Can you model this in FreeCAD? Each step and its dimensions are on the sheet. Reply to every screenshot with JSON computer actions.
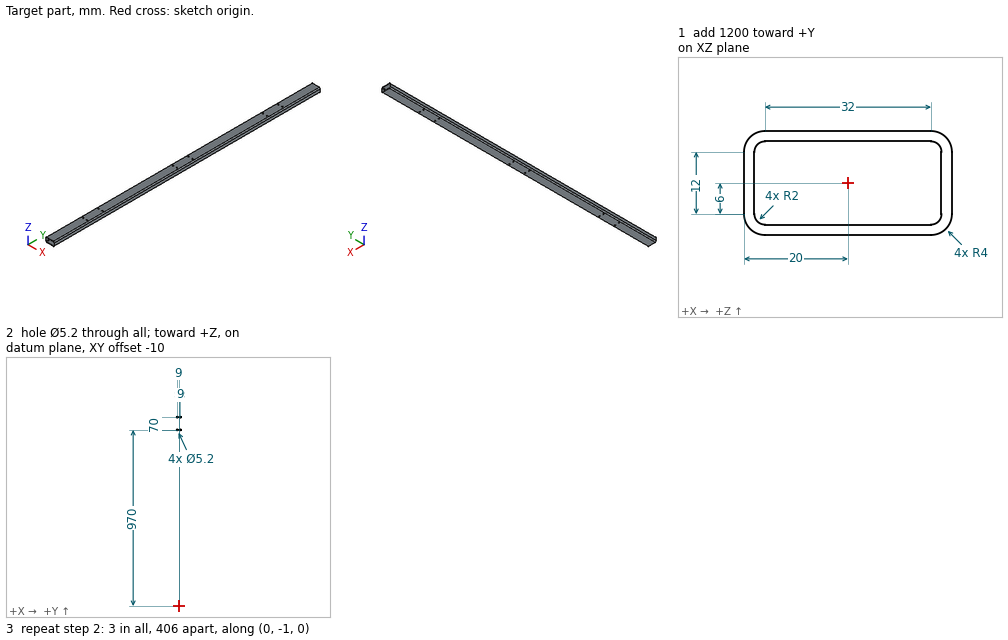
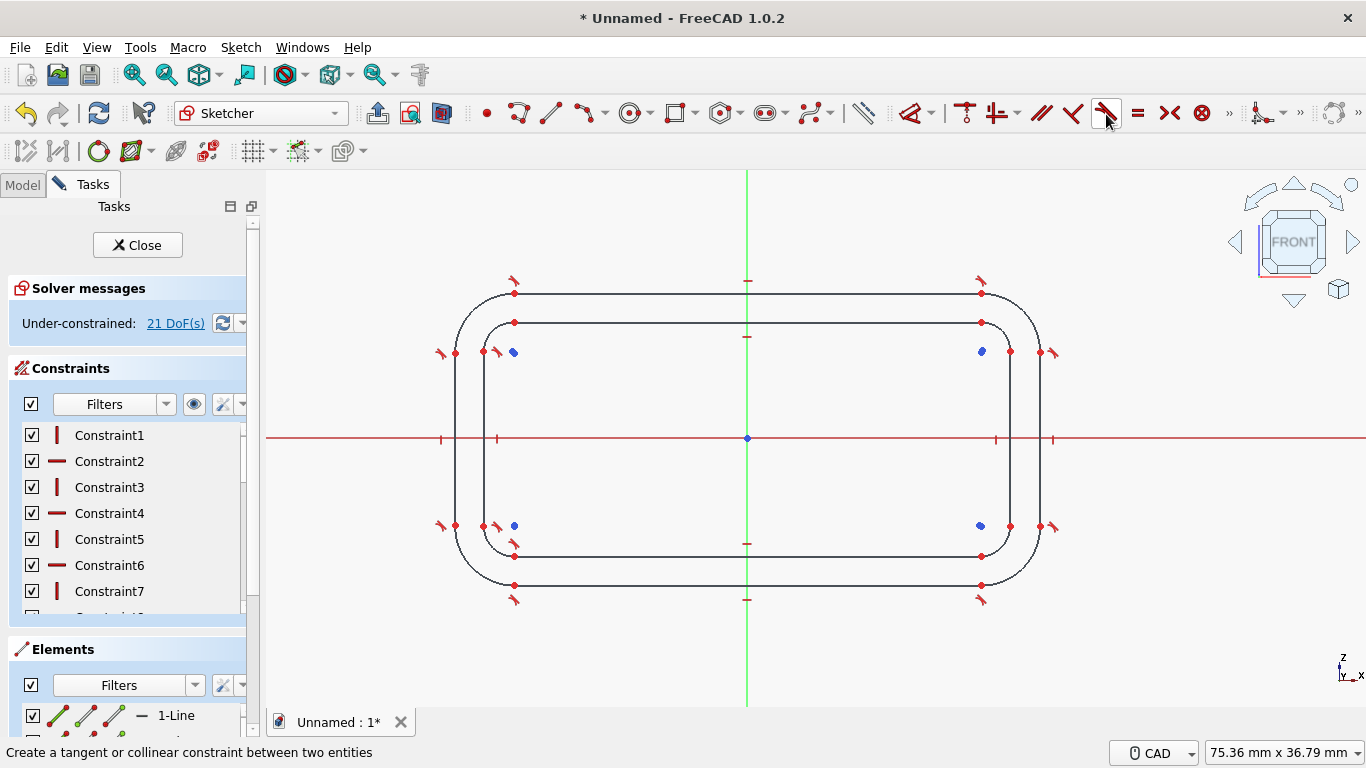
{"action": "left_click", "coordinate": [654, 557]}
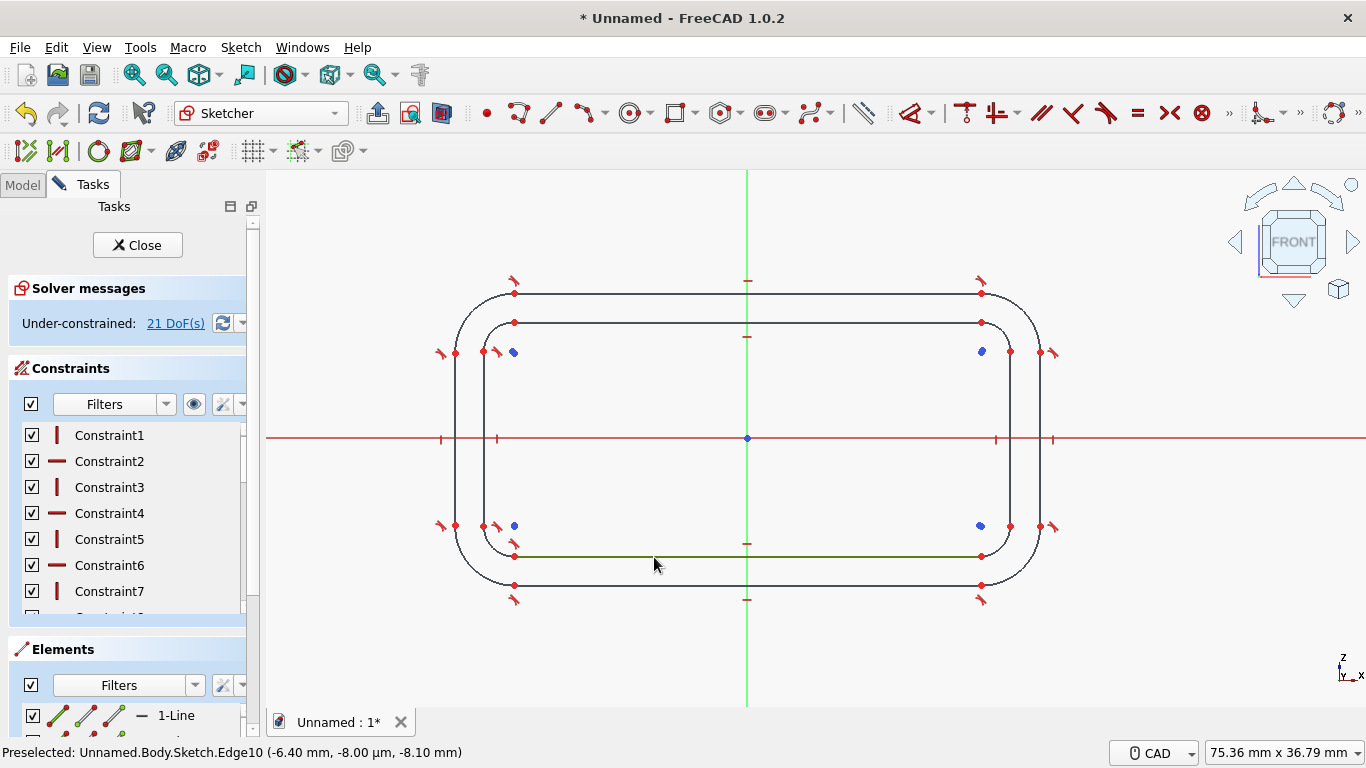
{"action": "left_click", "coordinate": [994, 553]}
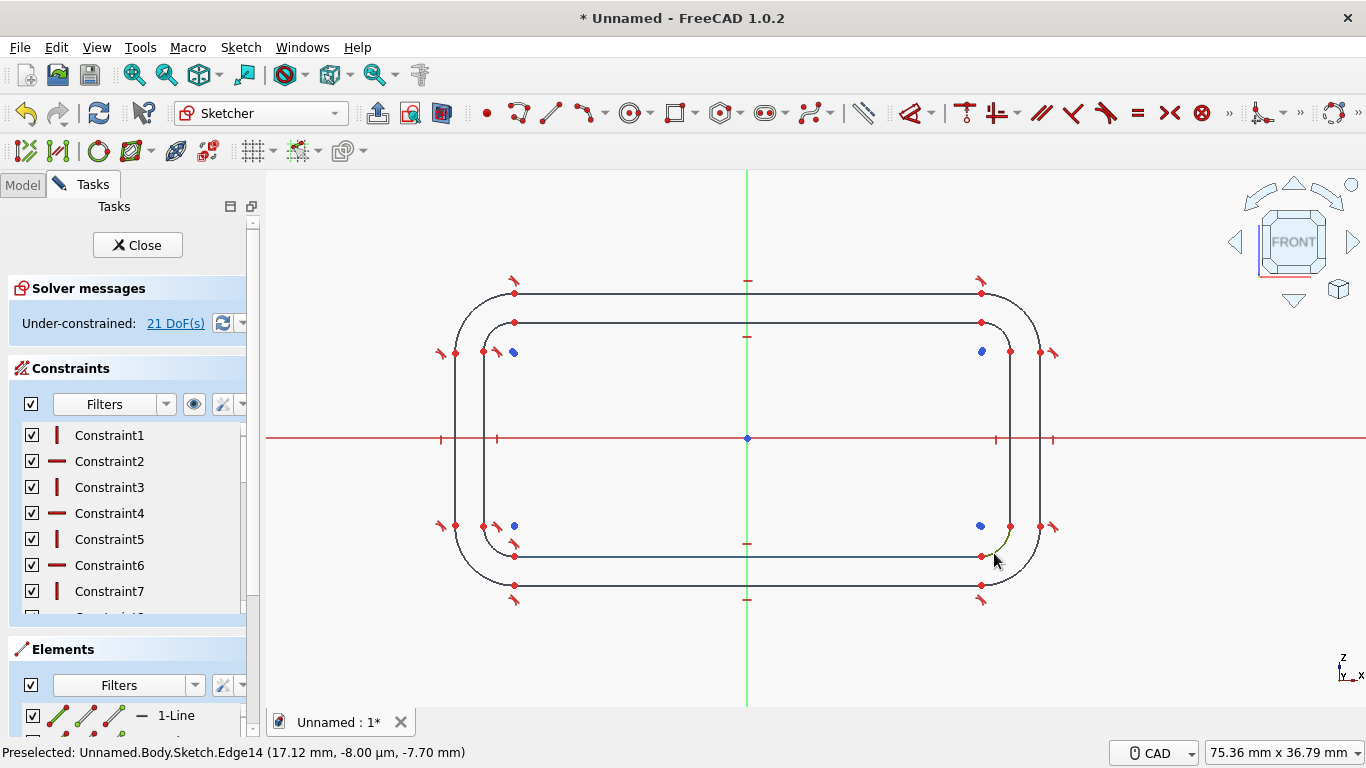
{"action": "left_click", "coordinate": [1106, 114]}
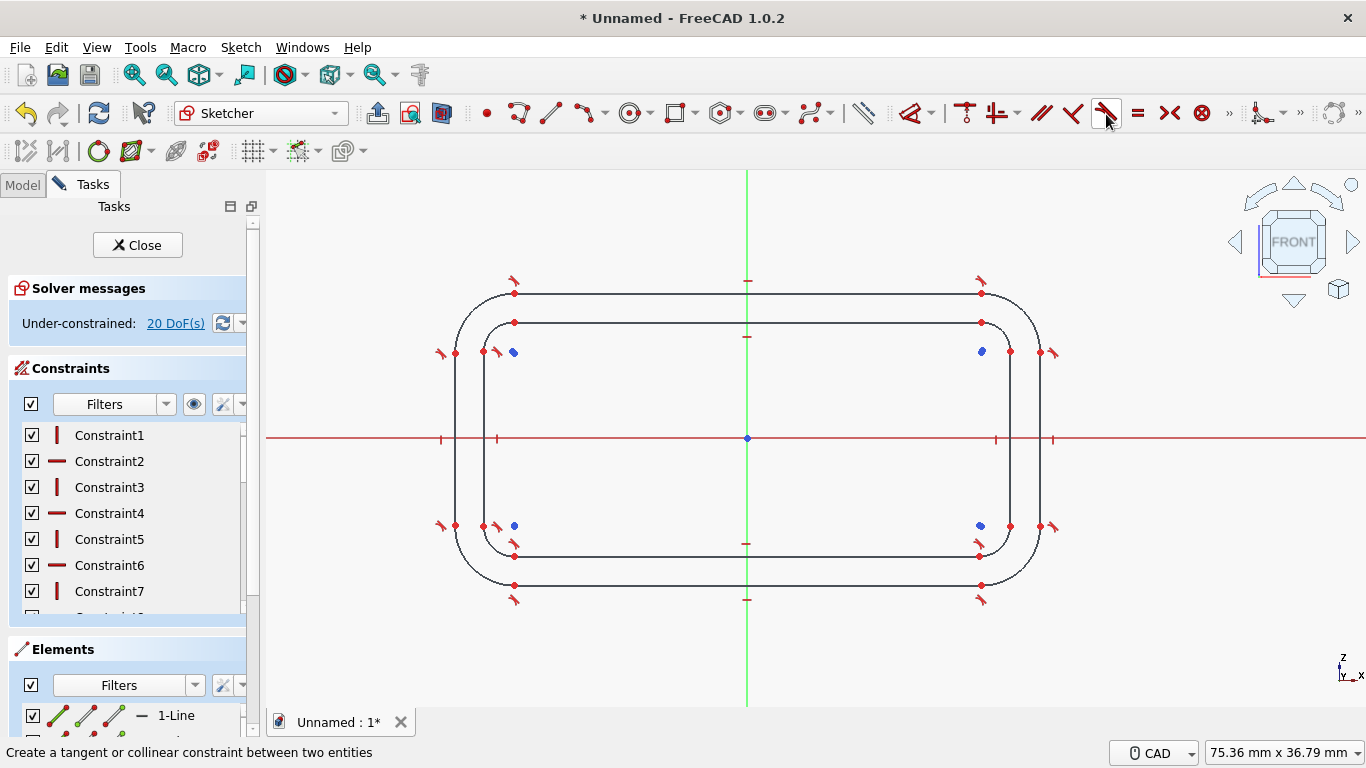
{"action": "left_click", "coordinate": [1010, 474]}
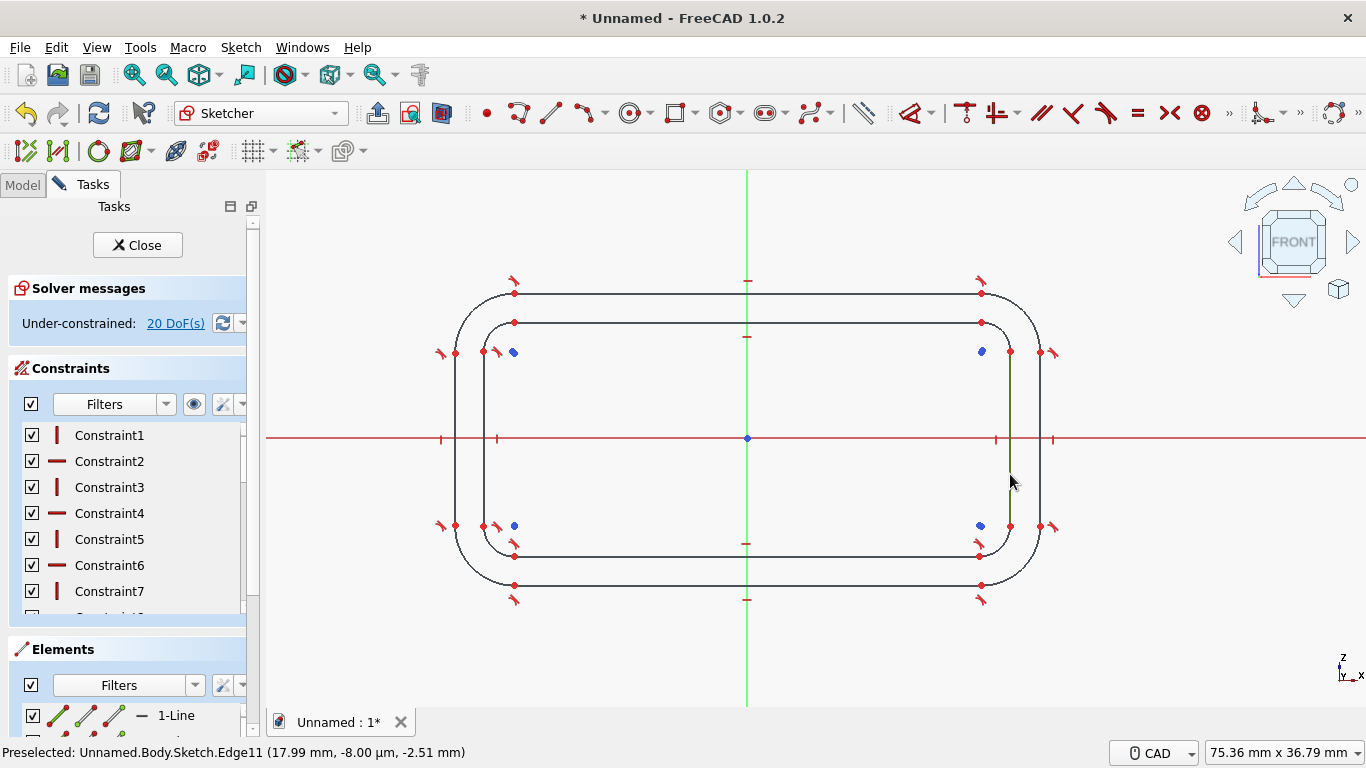
{"action": "left_click", "coordinate": [993, 553]}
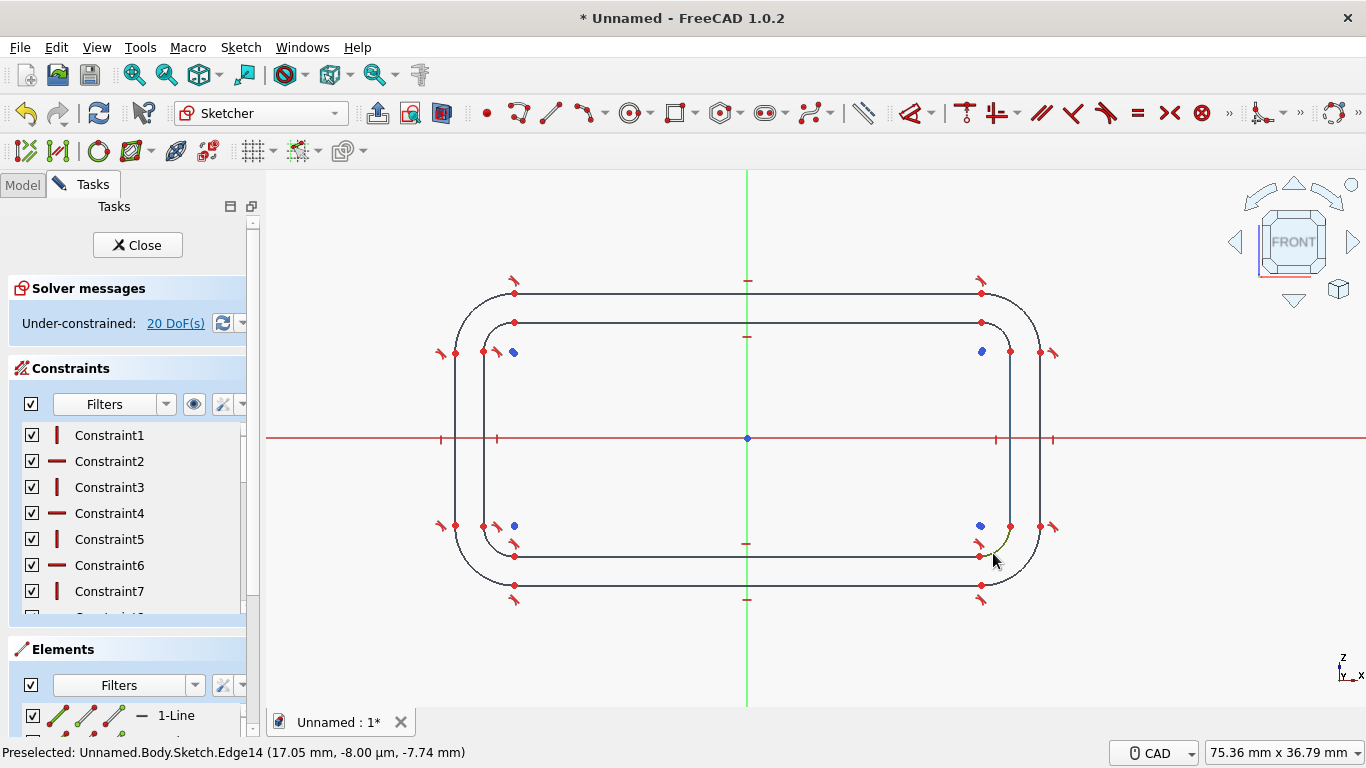
{"action": "left_click", "coordinate": [1106, 114]}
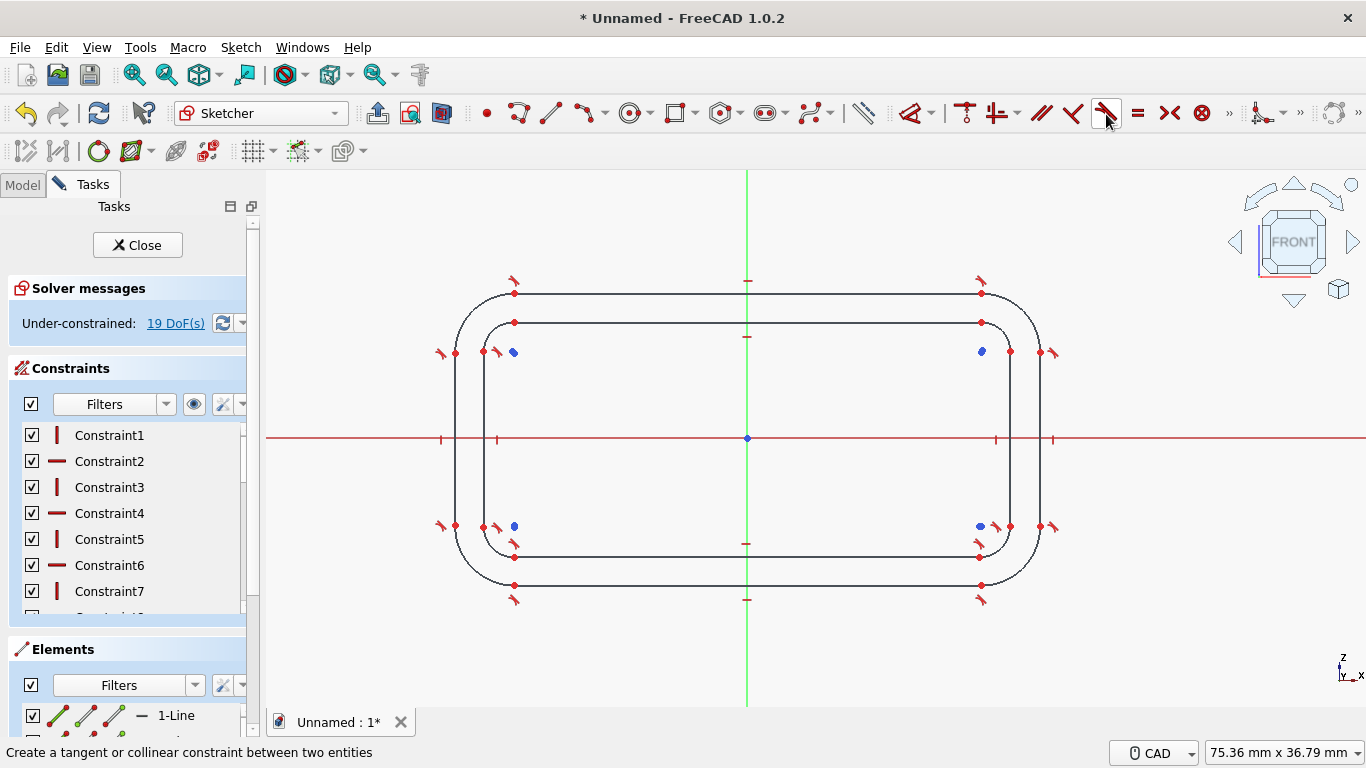
{"action": "left_click", "coordinate": [1010, 474]}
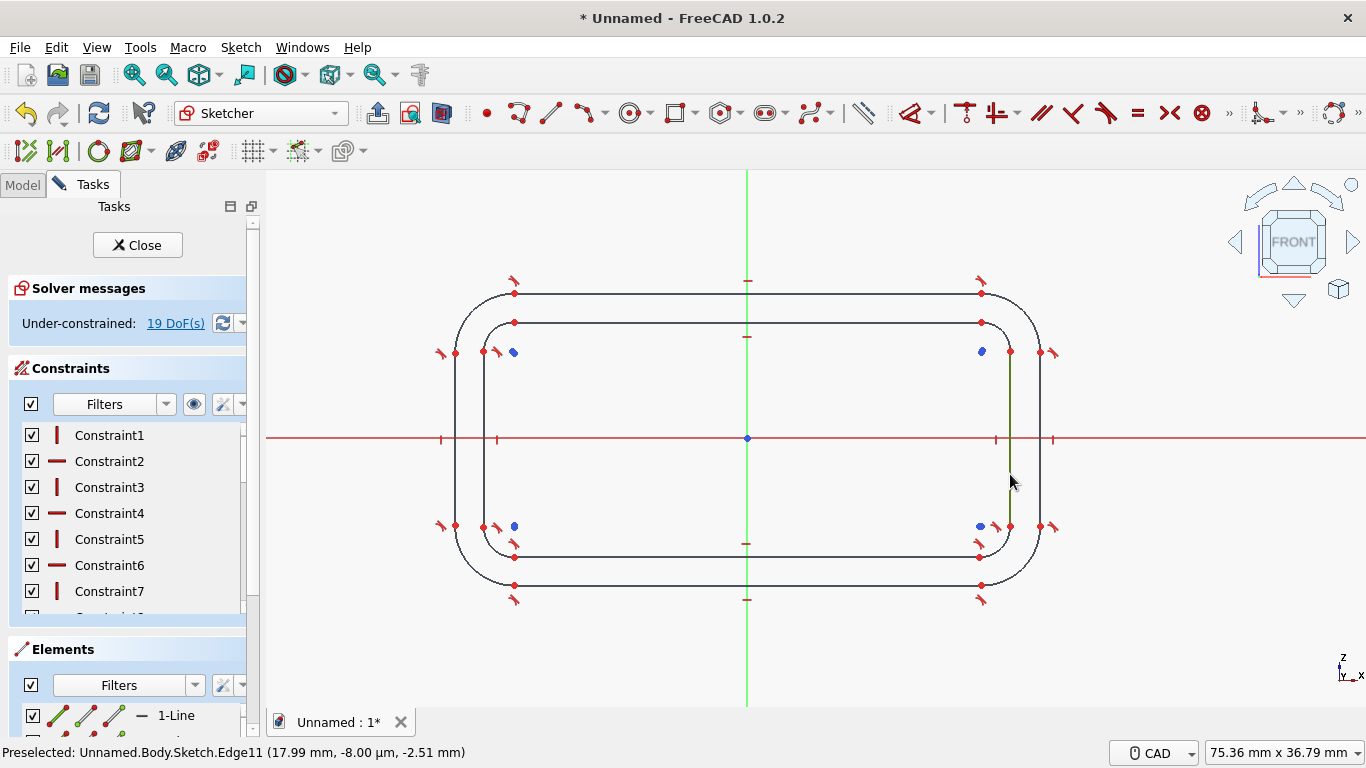
{"action": "left_click", "coordinate": [1007, 338]}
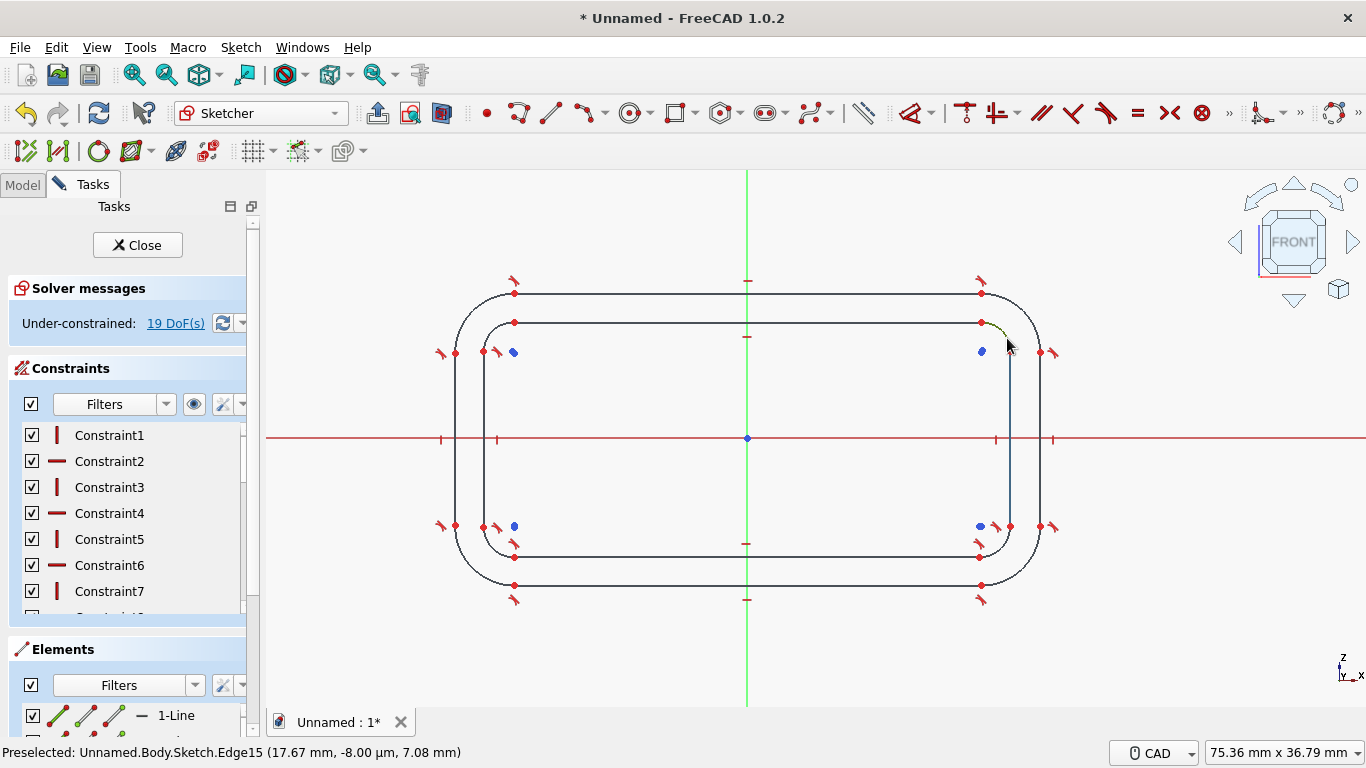
{"action": "left_click", "coordinate": [1106, 114]}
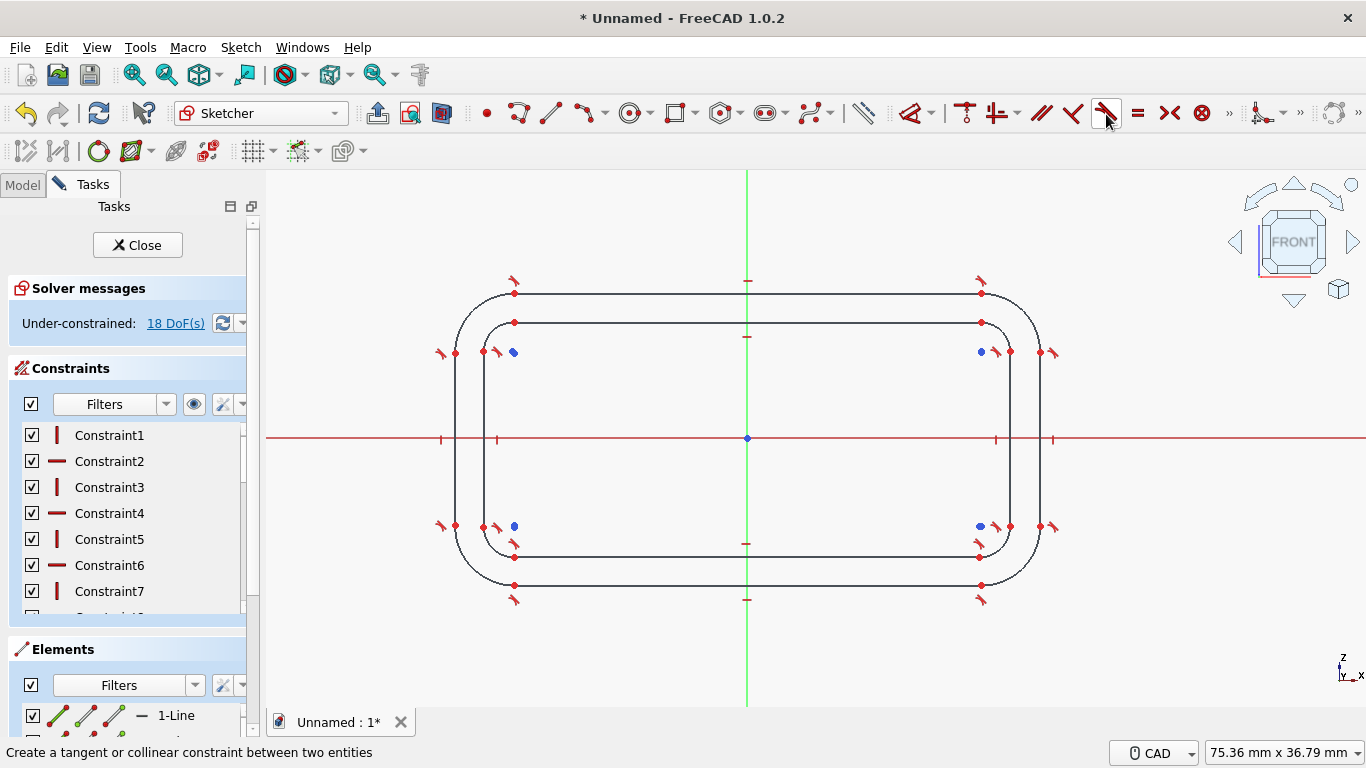
{"action": "left_click", "coordinate": [841, 323]}